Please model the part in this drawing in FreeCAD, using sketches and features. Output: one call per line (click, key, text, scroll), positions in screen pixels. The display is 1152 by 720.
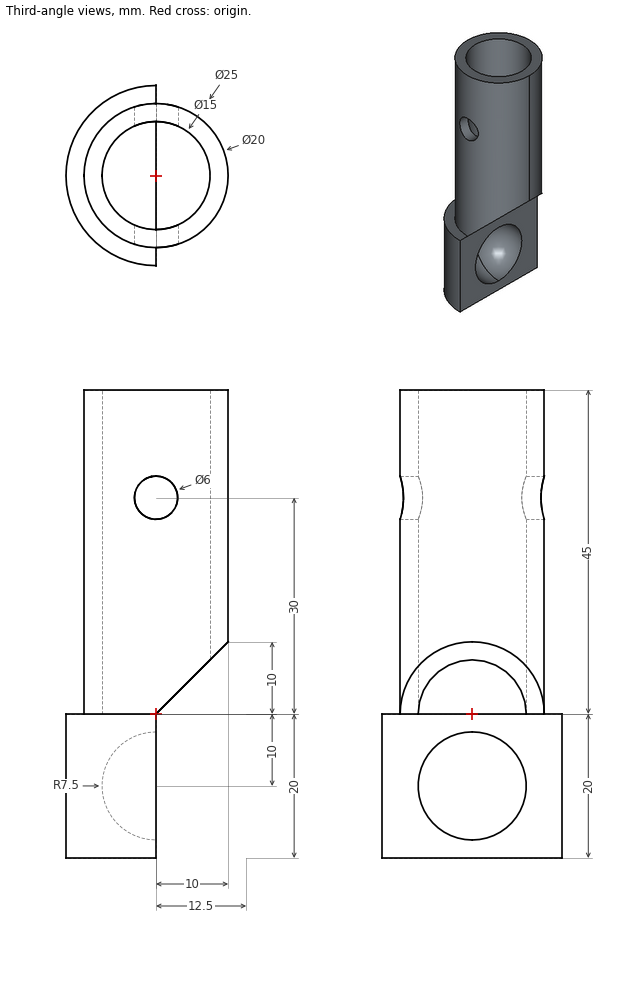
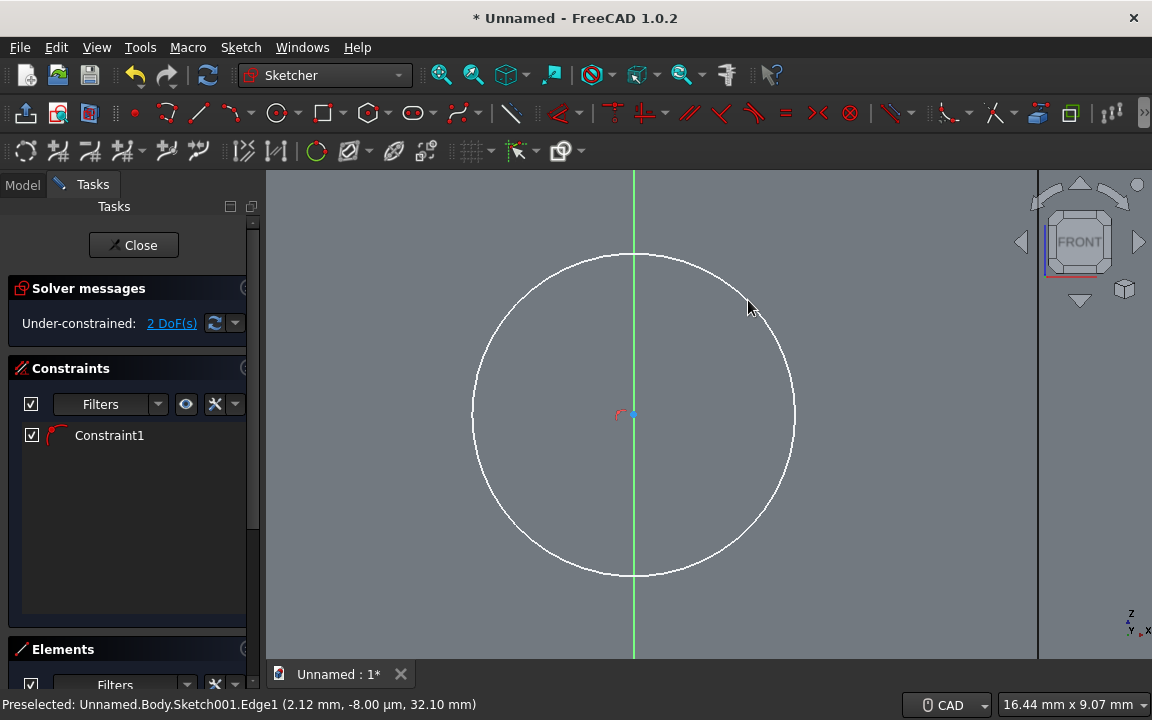
click(558, 114)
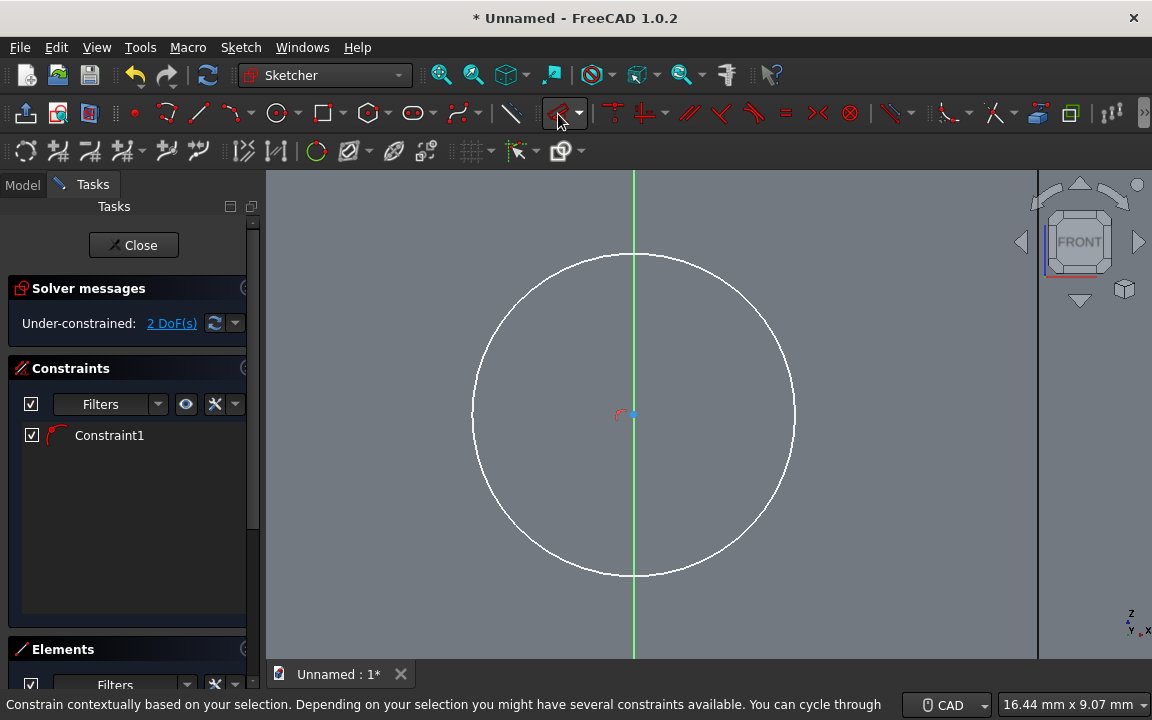
click(748, 301)
click(771, 278)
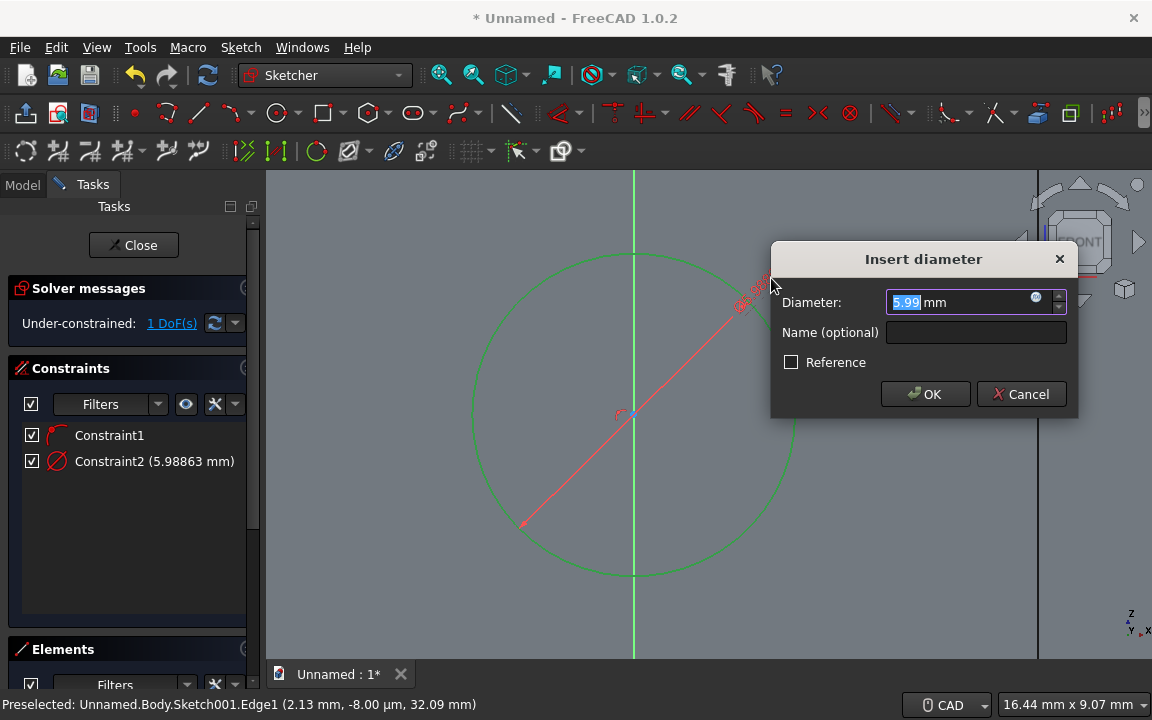
text(6)
key(Return)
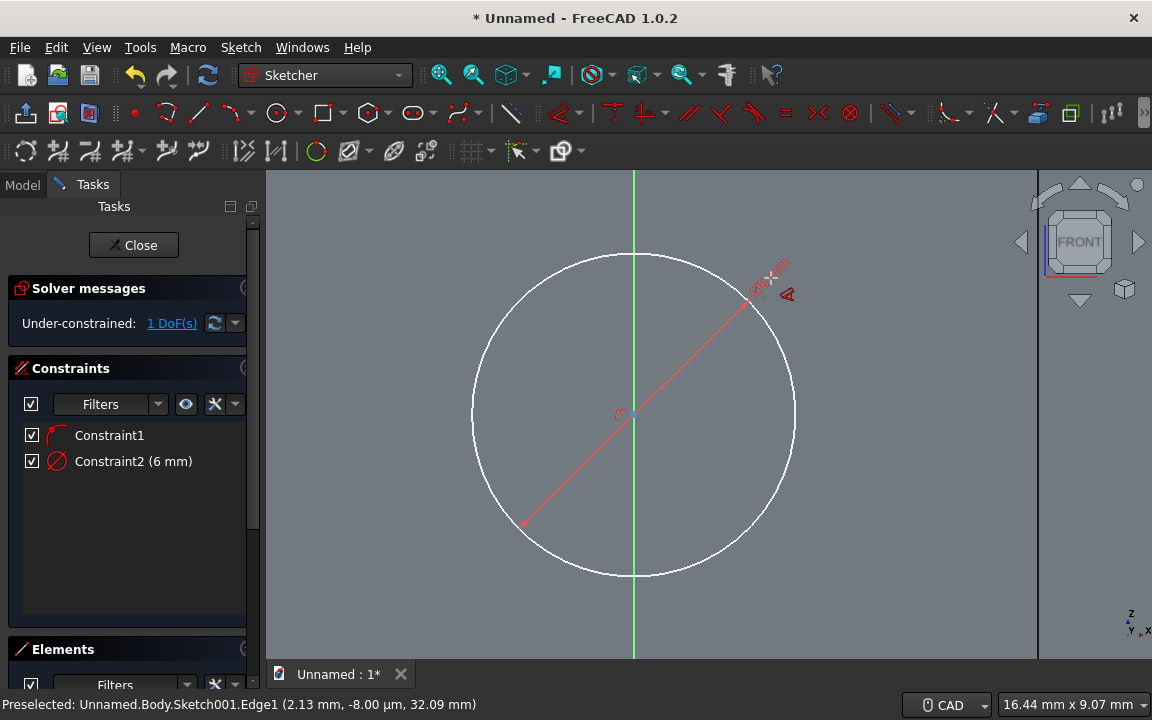
click(634, 415)
click(668, 523)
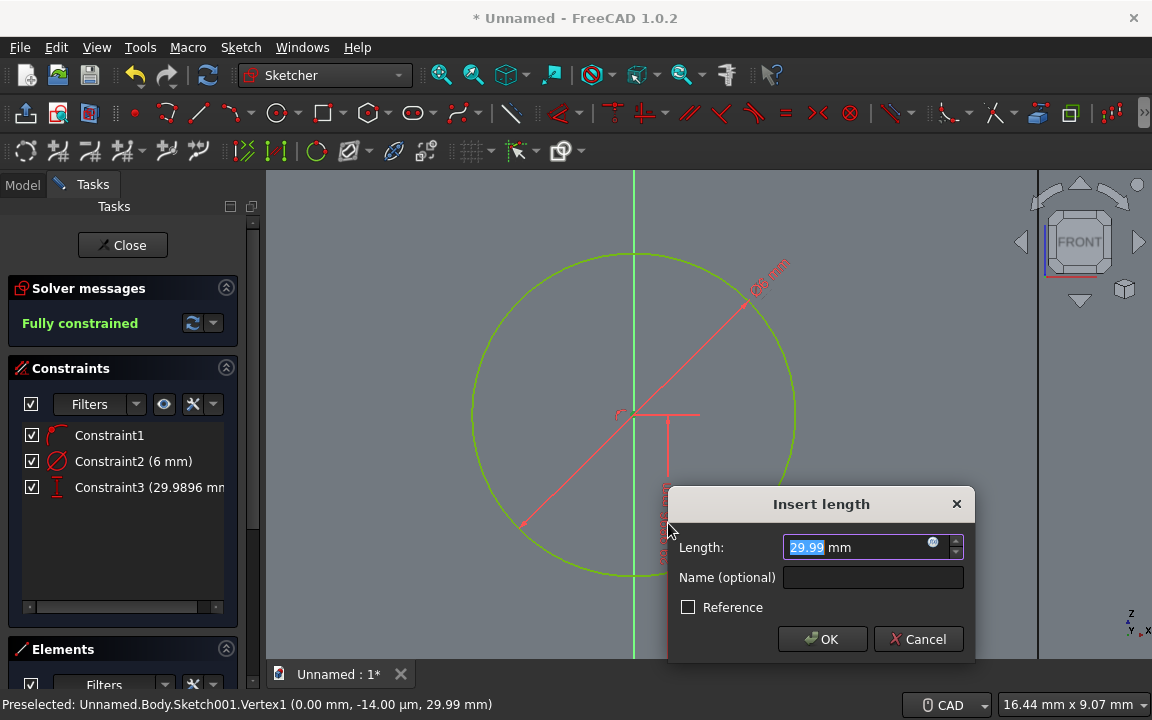
text(30)
key(Return)
key(Escape)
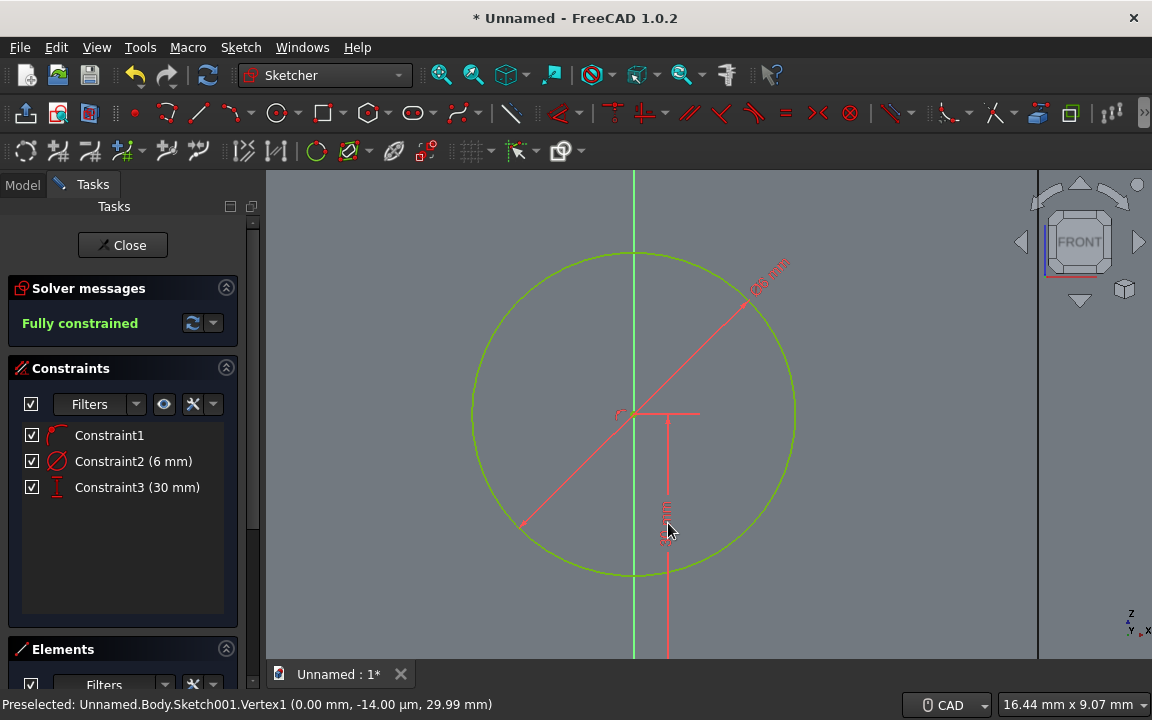
click(123, 245)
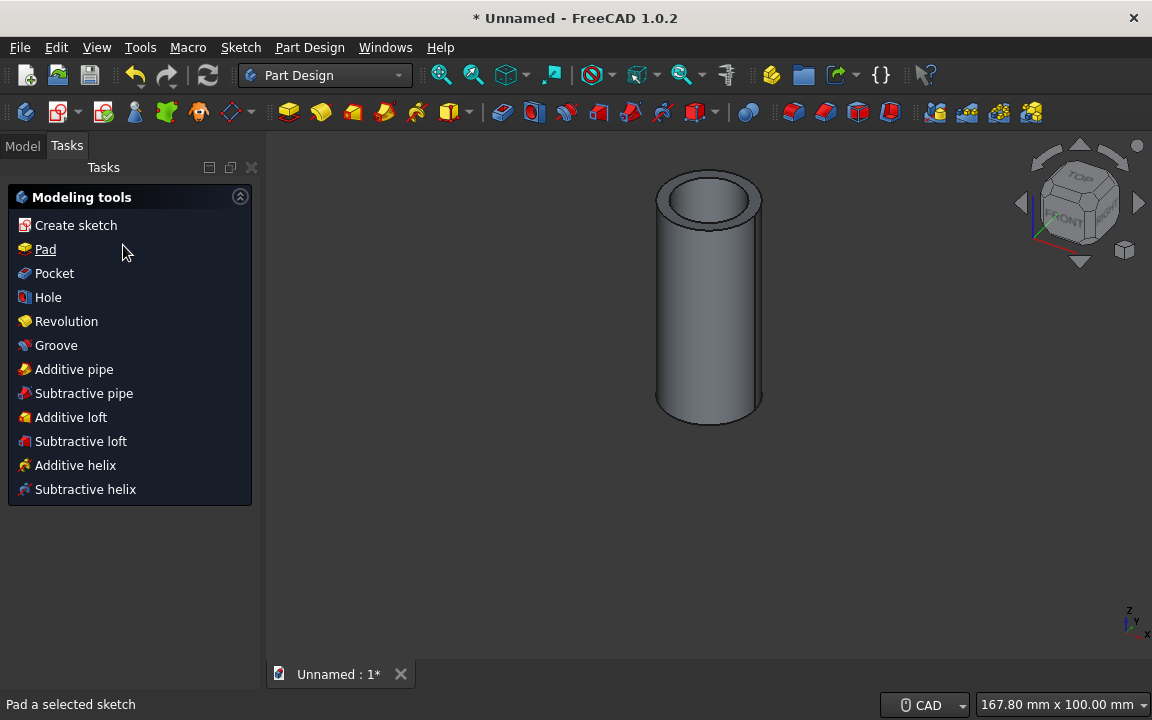
click(504, 112)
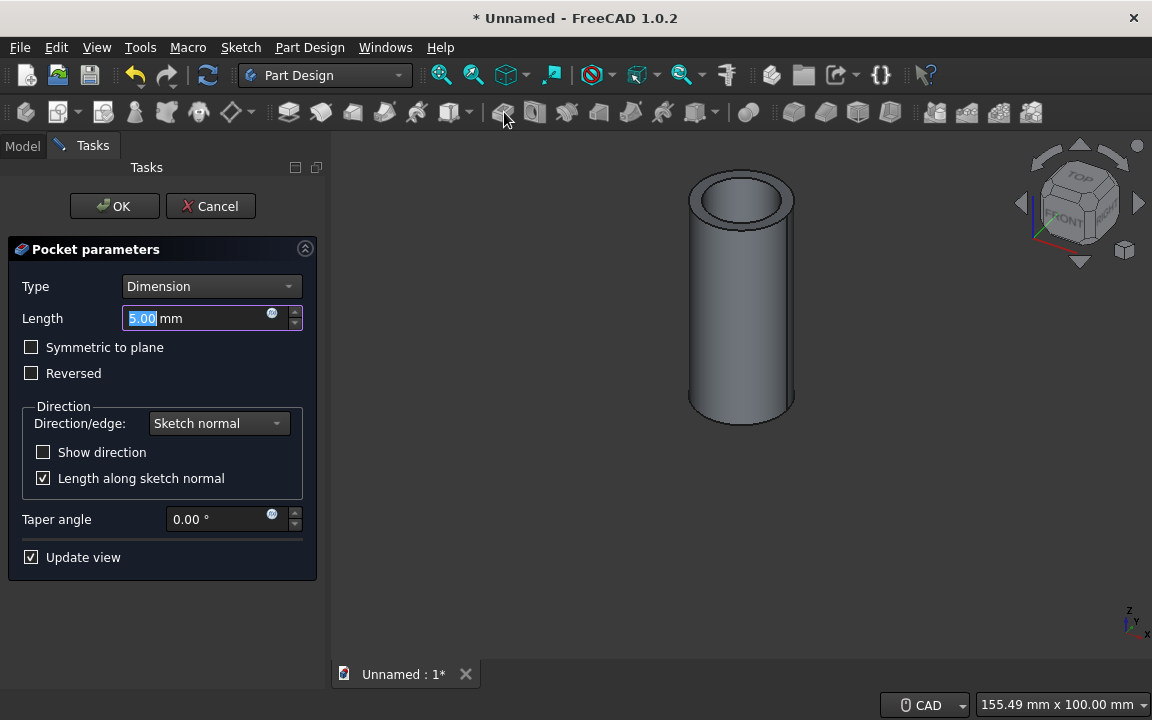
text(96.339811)
key(Tab)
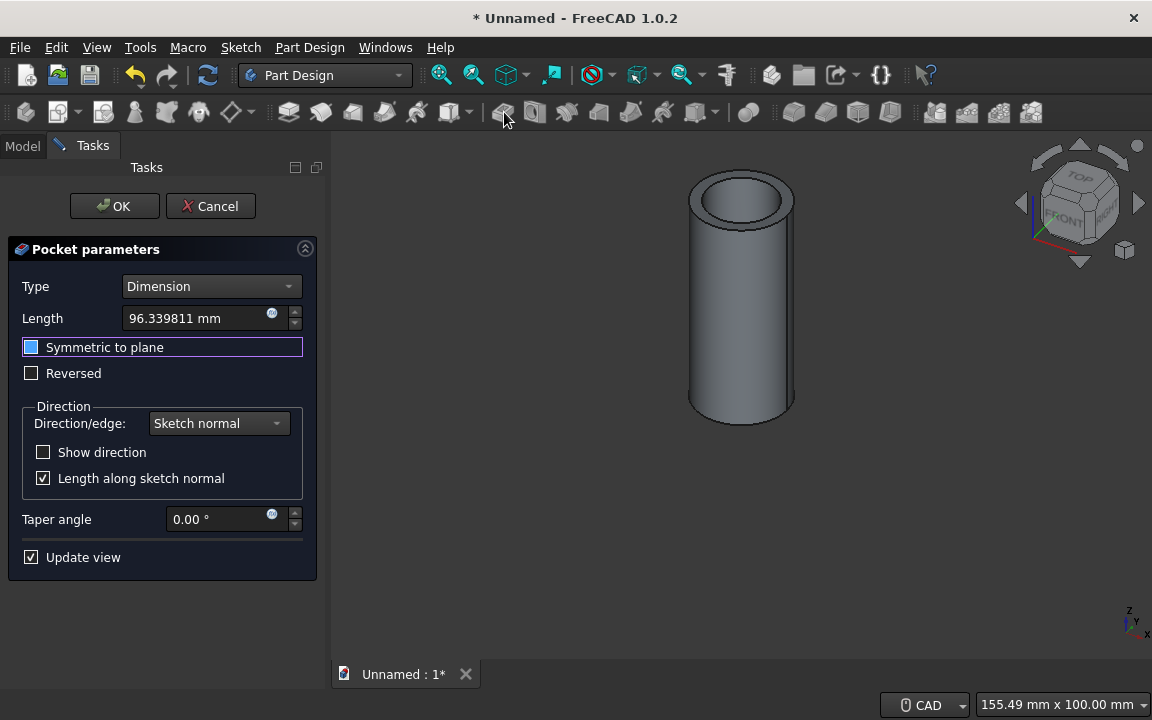
click(30, 347)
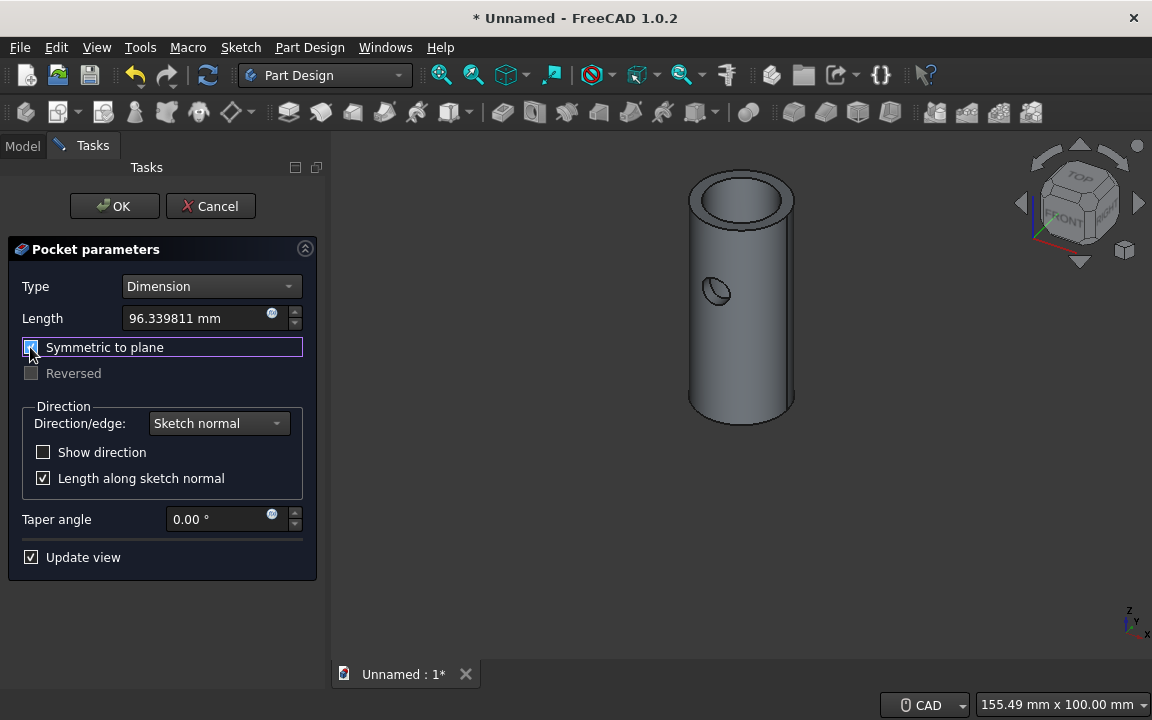
click(115, 206)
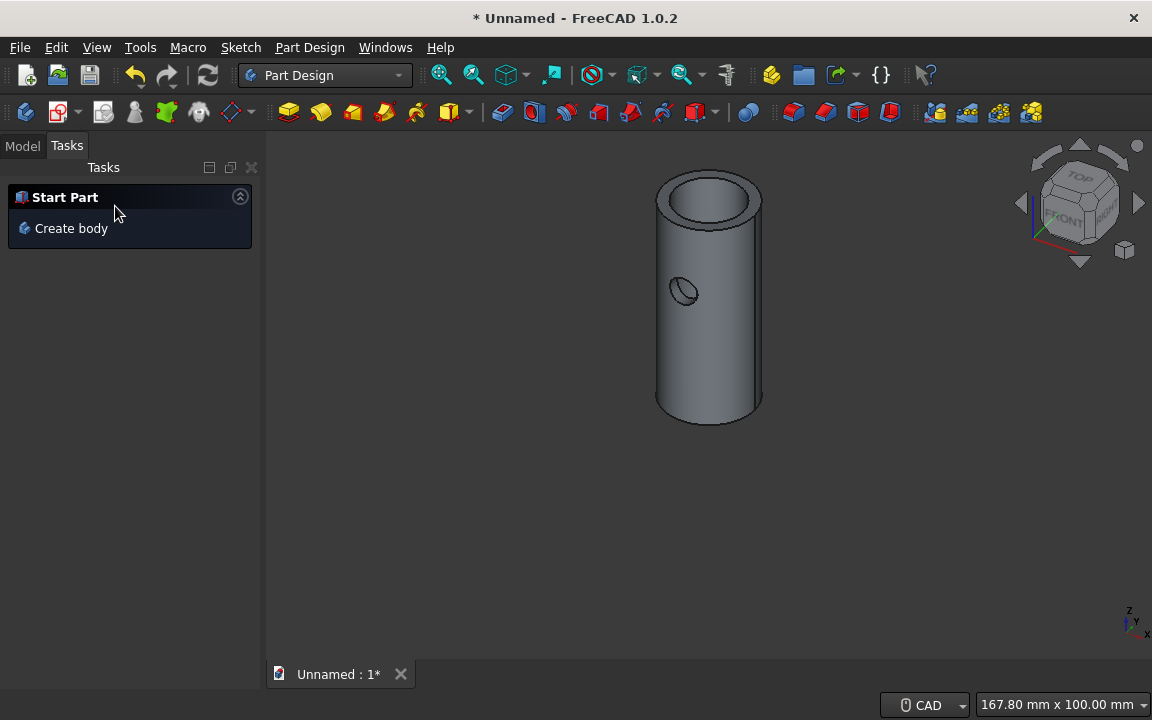
click(58, 112)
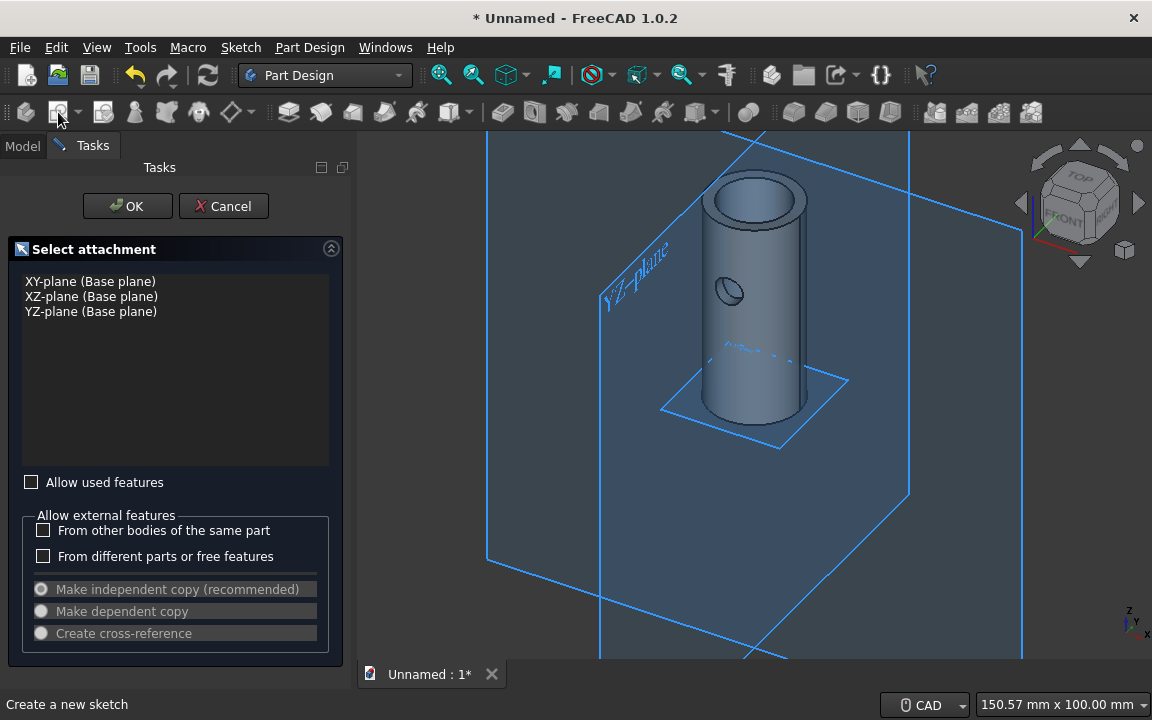
click(82, 282)